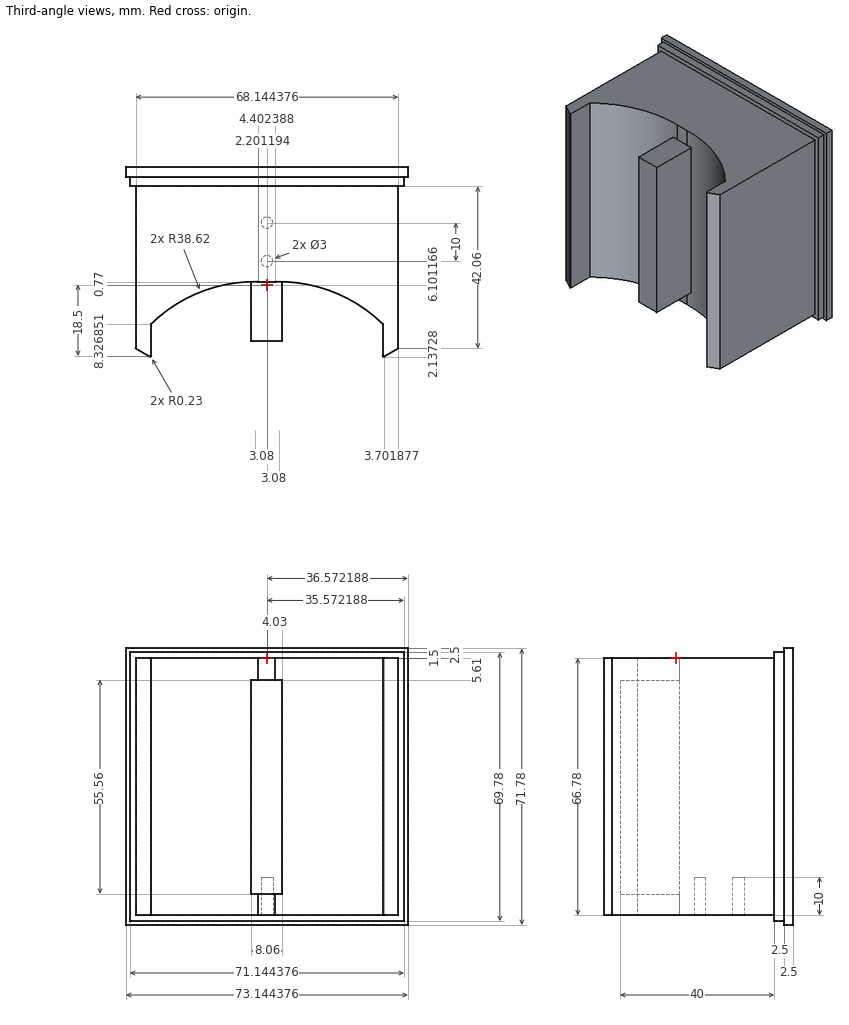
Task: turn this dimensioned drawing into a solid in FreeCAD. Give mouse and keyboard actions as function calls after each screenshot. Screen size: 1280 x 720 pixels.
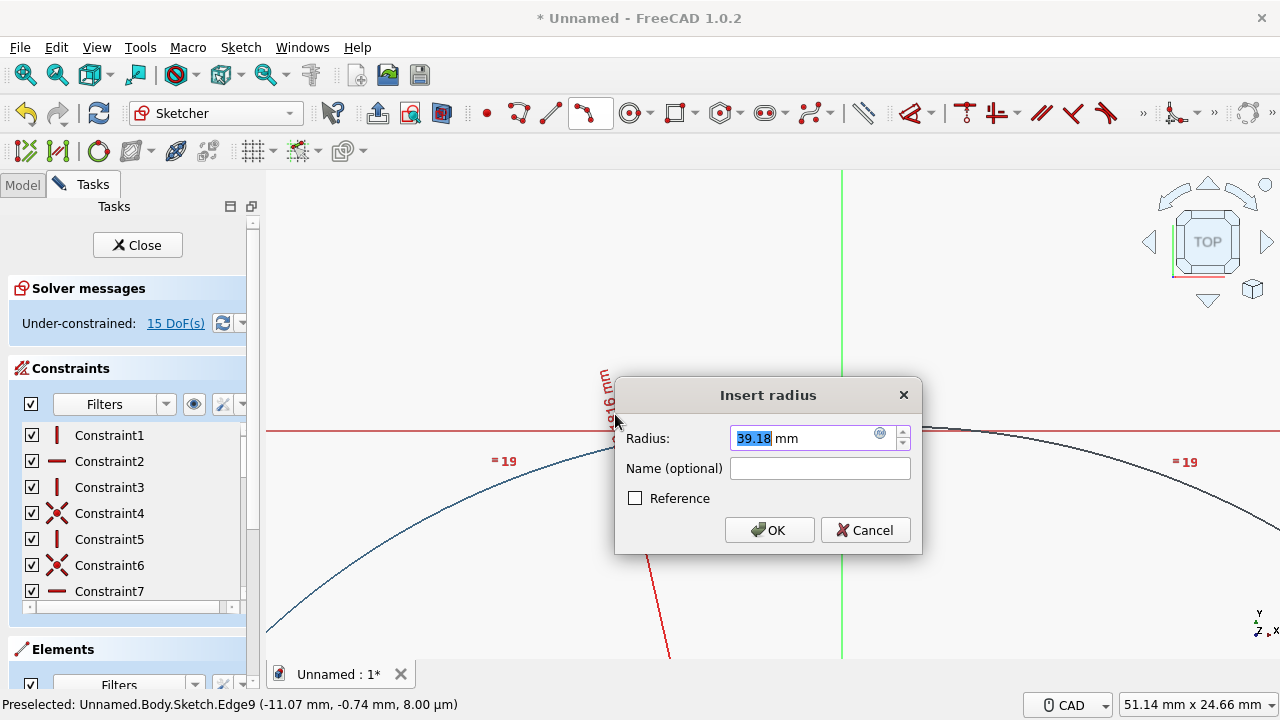
text(38.62)
key(Return)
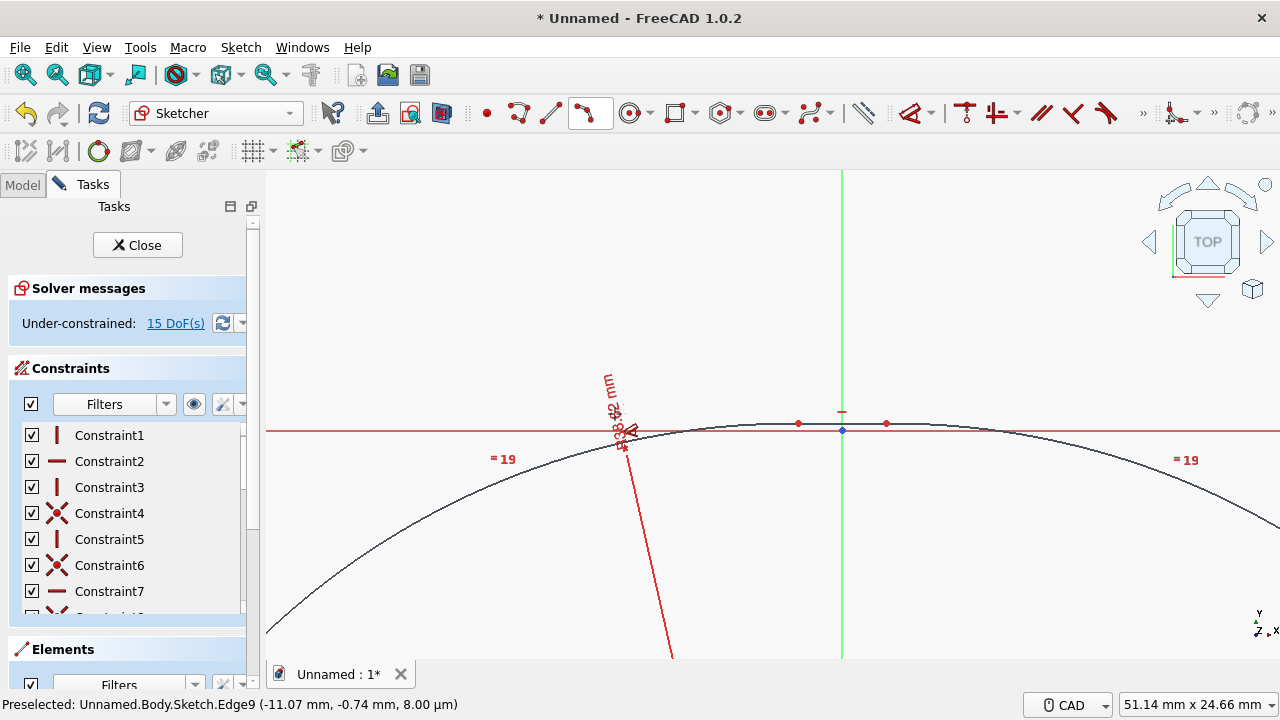
scroll(624, 444, down, 5)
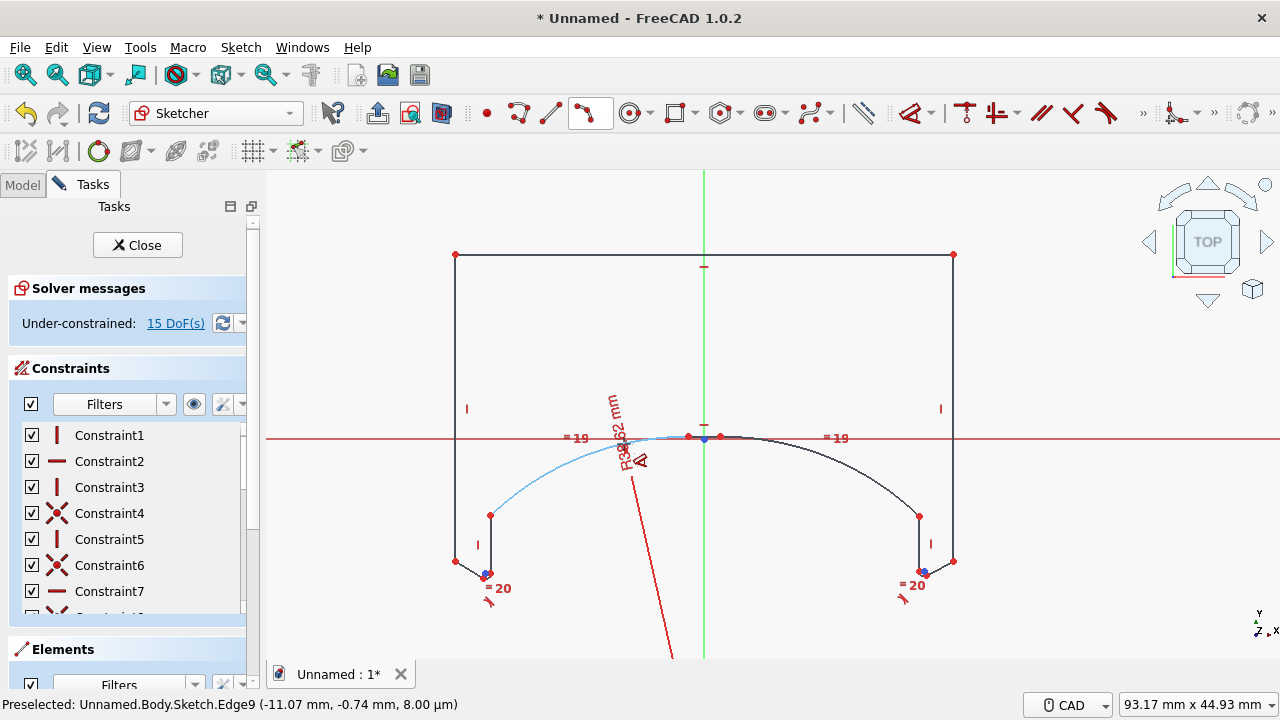
scroll(922, 576, up, 16)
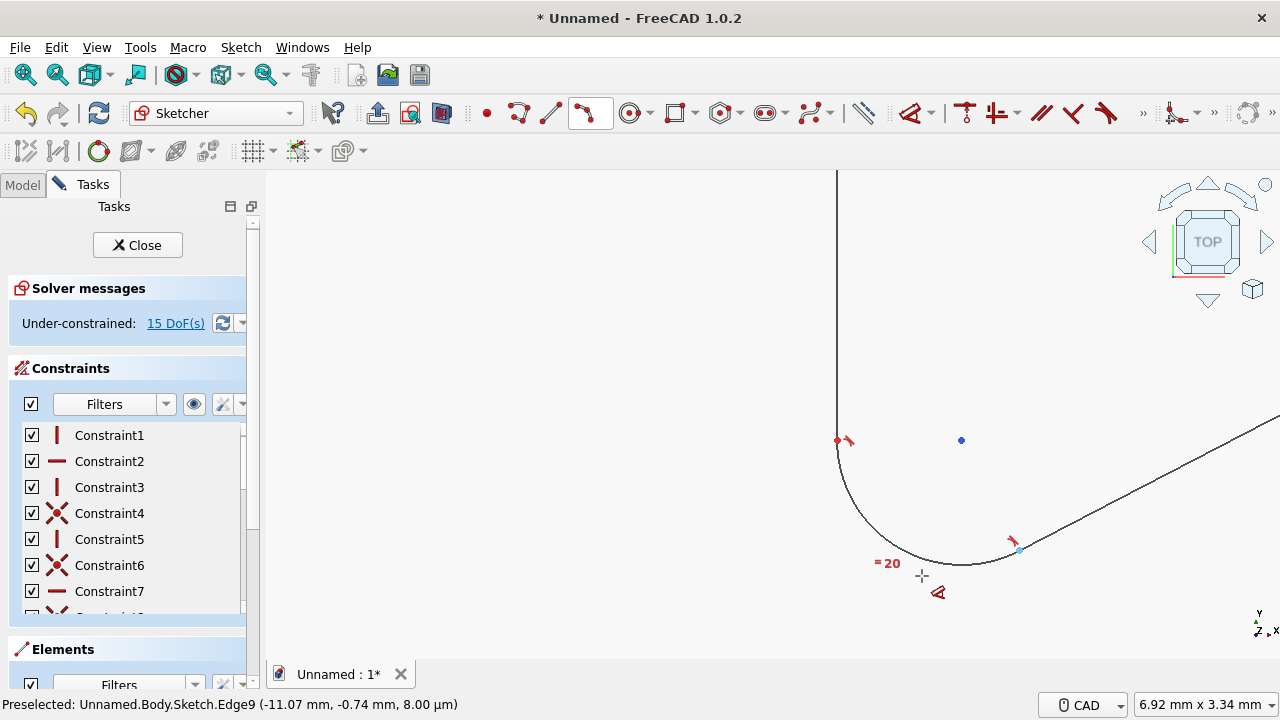
click(897, 547)
click(880, 574)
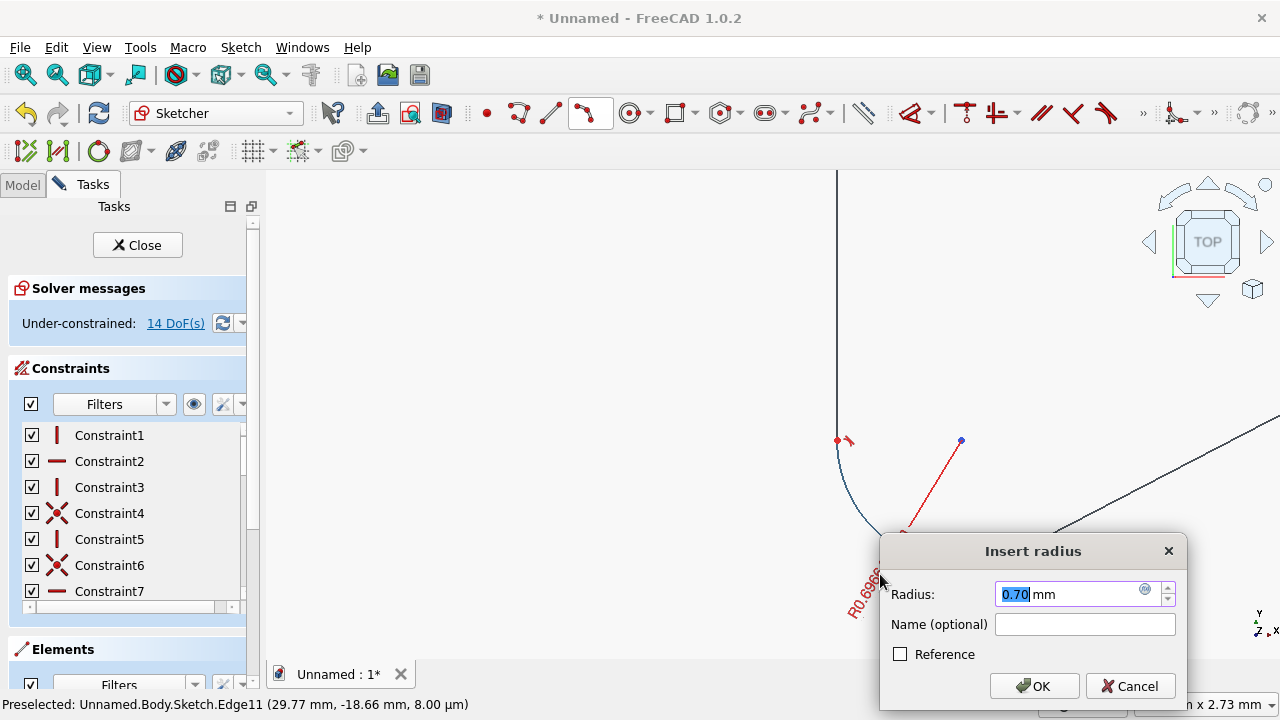
text(0.23)
key(Return)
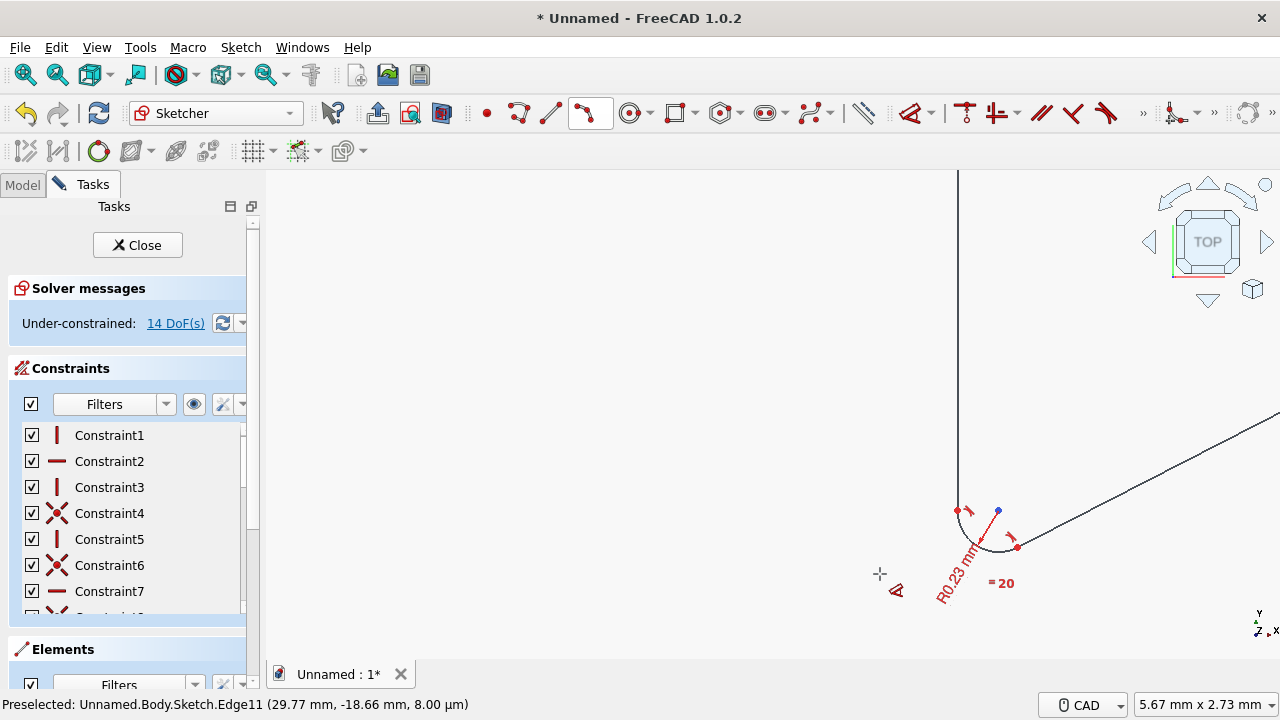
scroll(923, 577, down, 16)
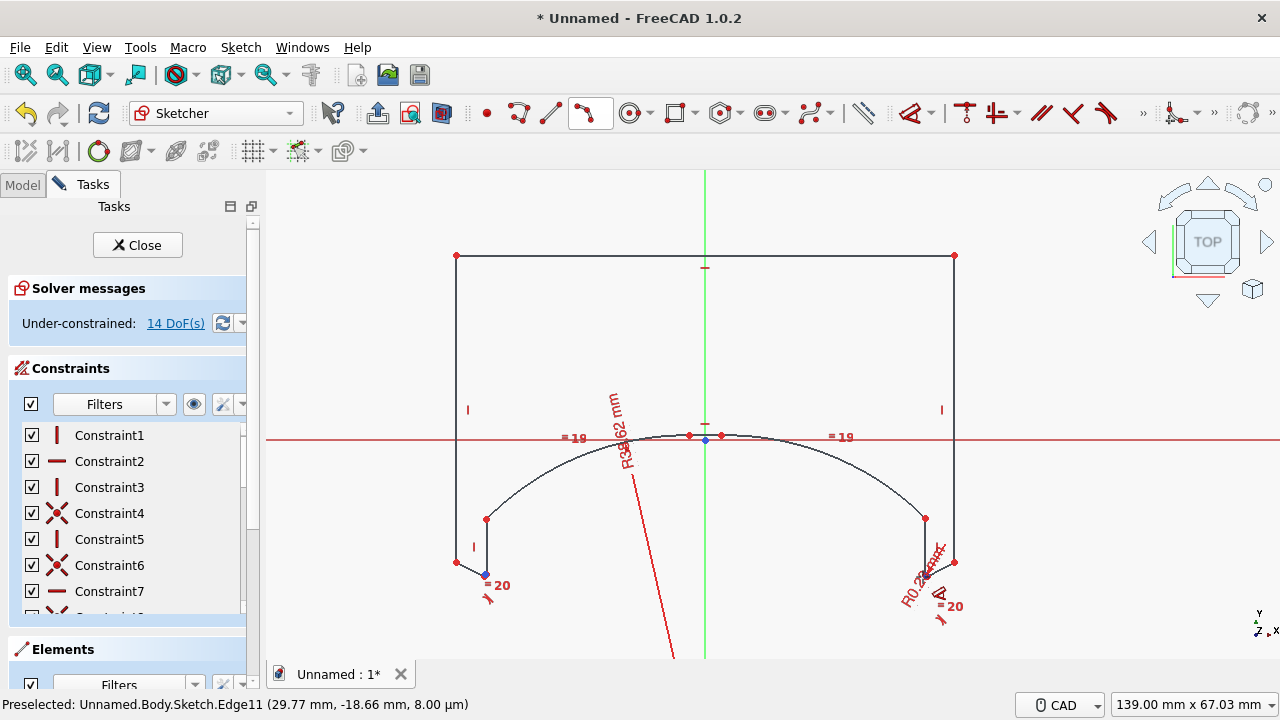
click(954, 471)
click(988, 409)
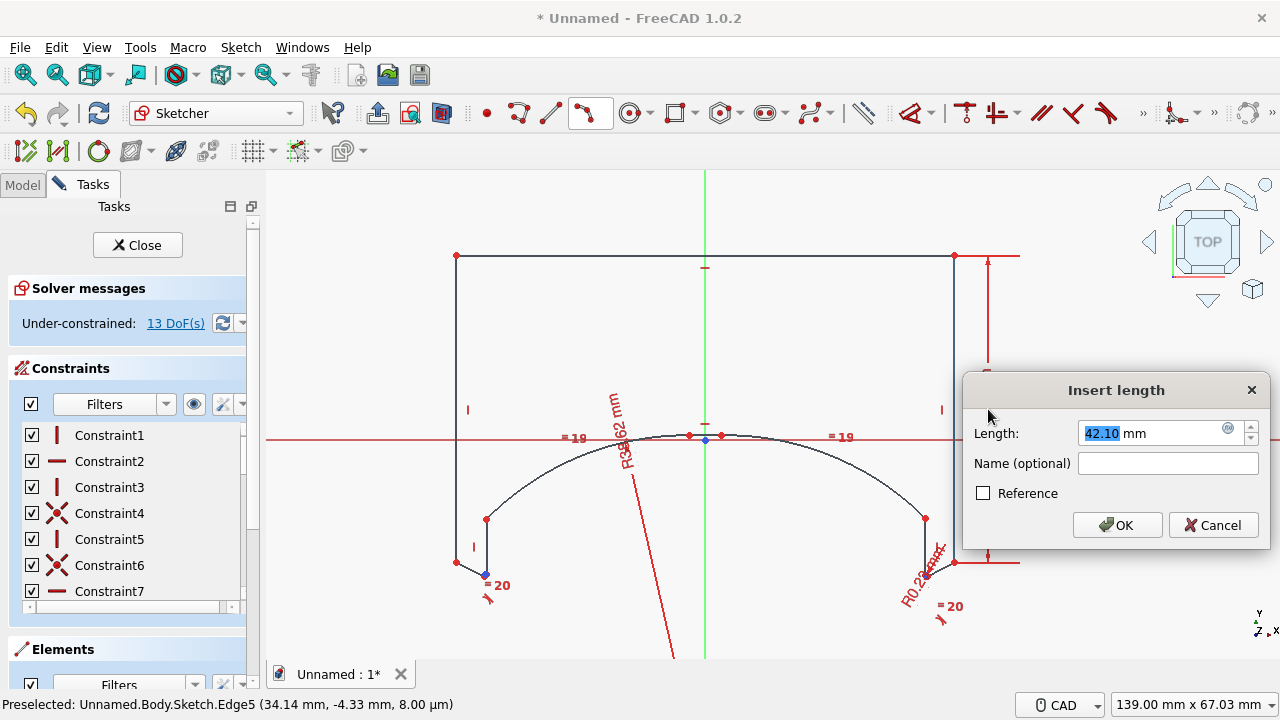
text(42.06)
key(Return)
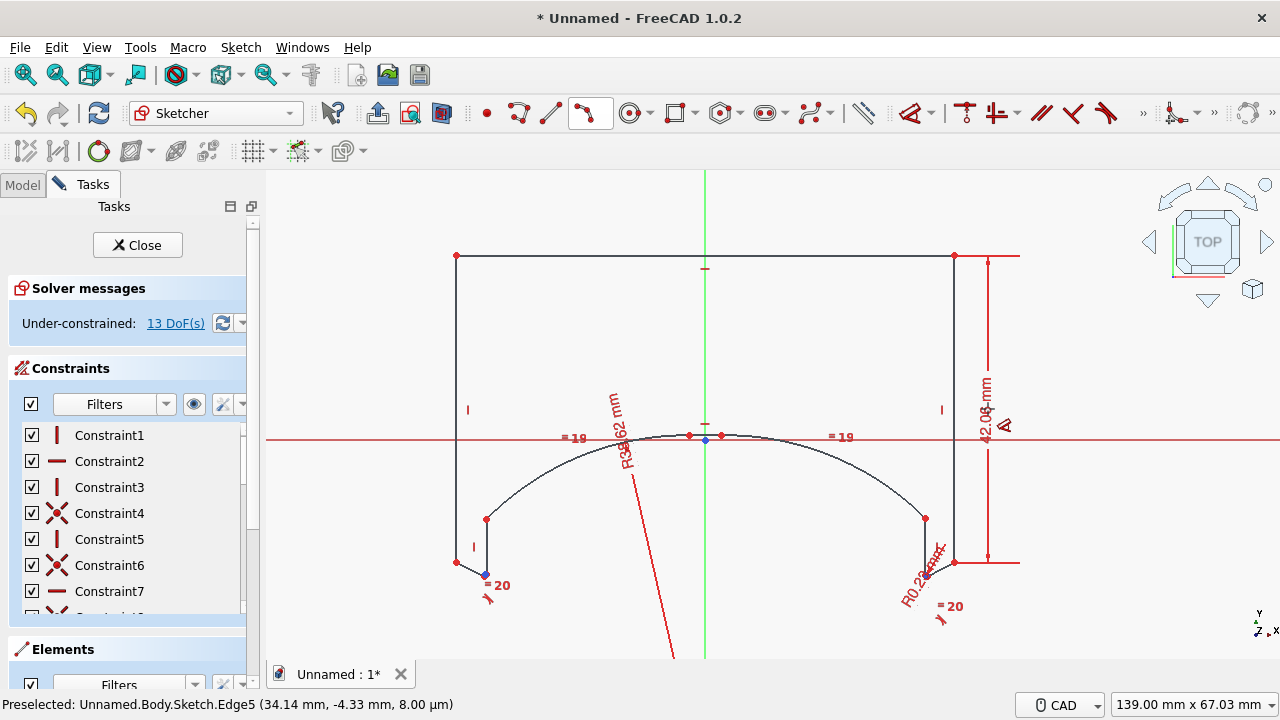
click(456, 348)
click(422, 409)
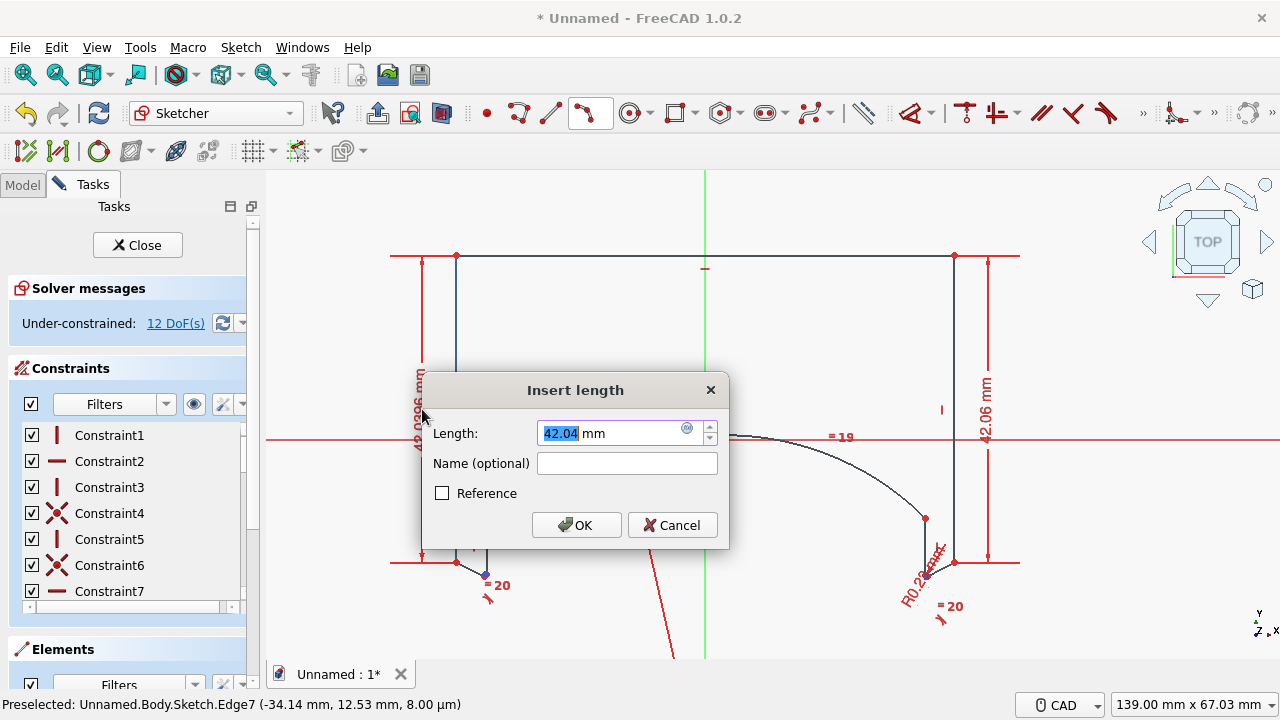
text(42.06)
key(Return)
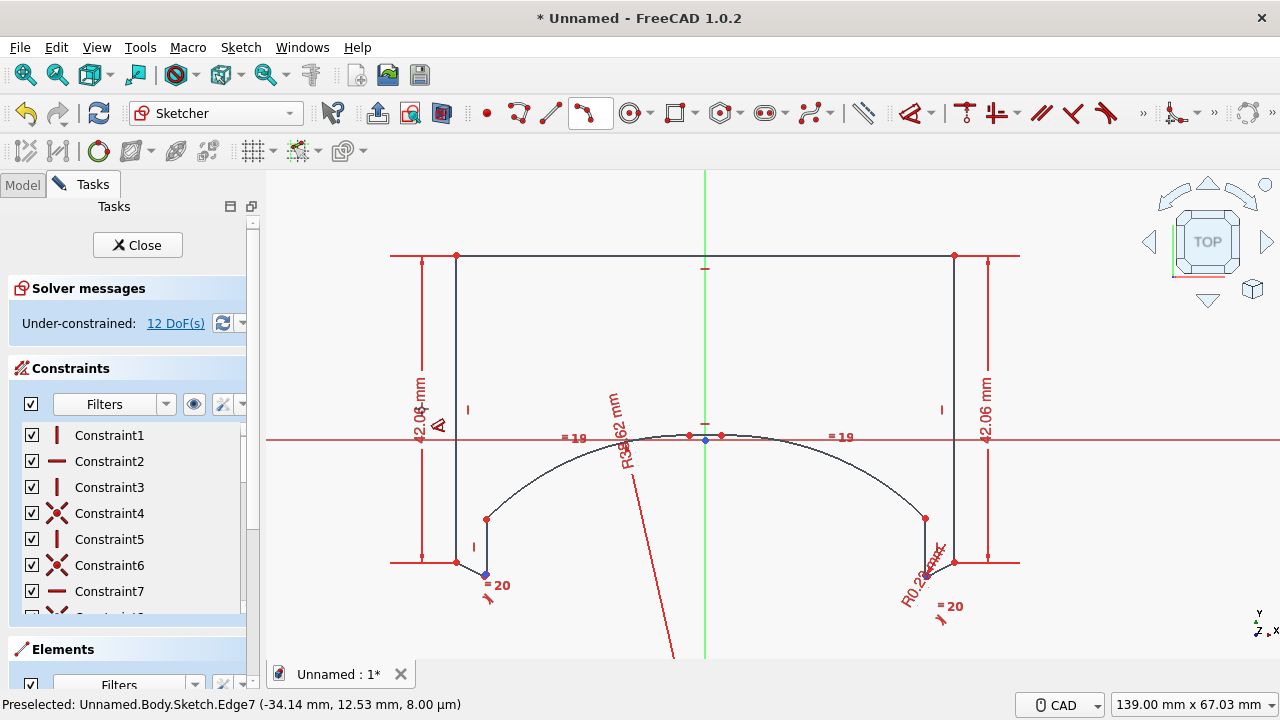
scroll(487, 575, up, 10)